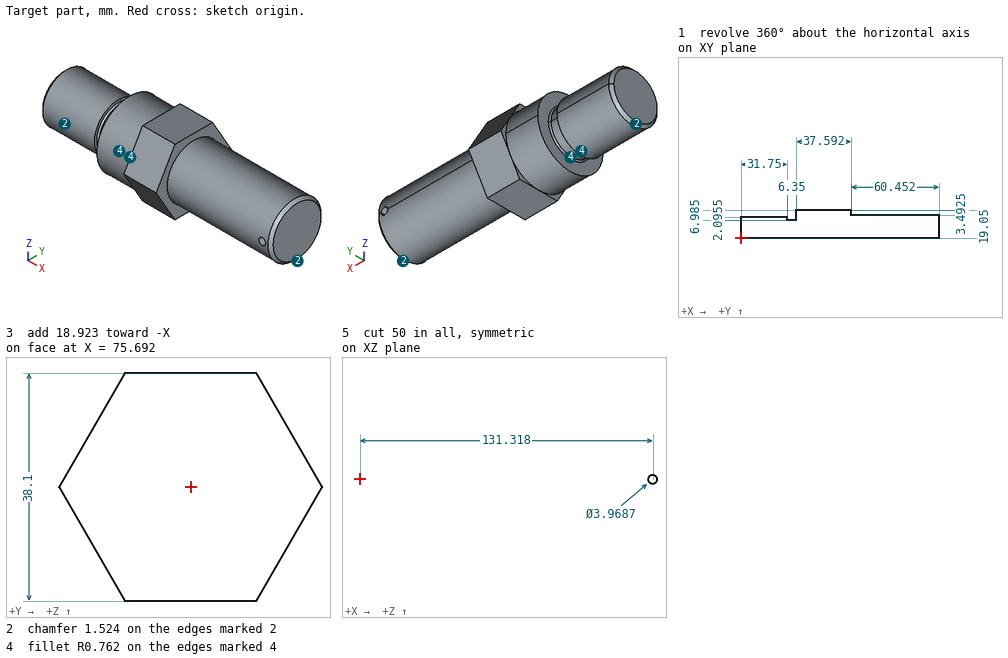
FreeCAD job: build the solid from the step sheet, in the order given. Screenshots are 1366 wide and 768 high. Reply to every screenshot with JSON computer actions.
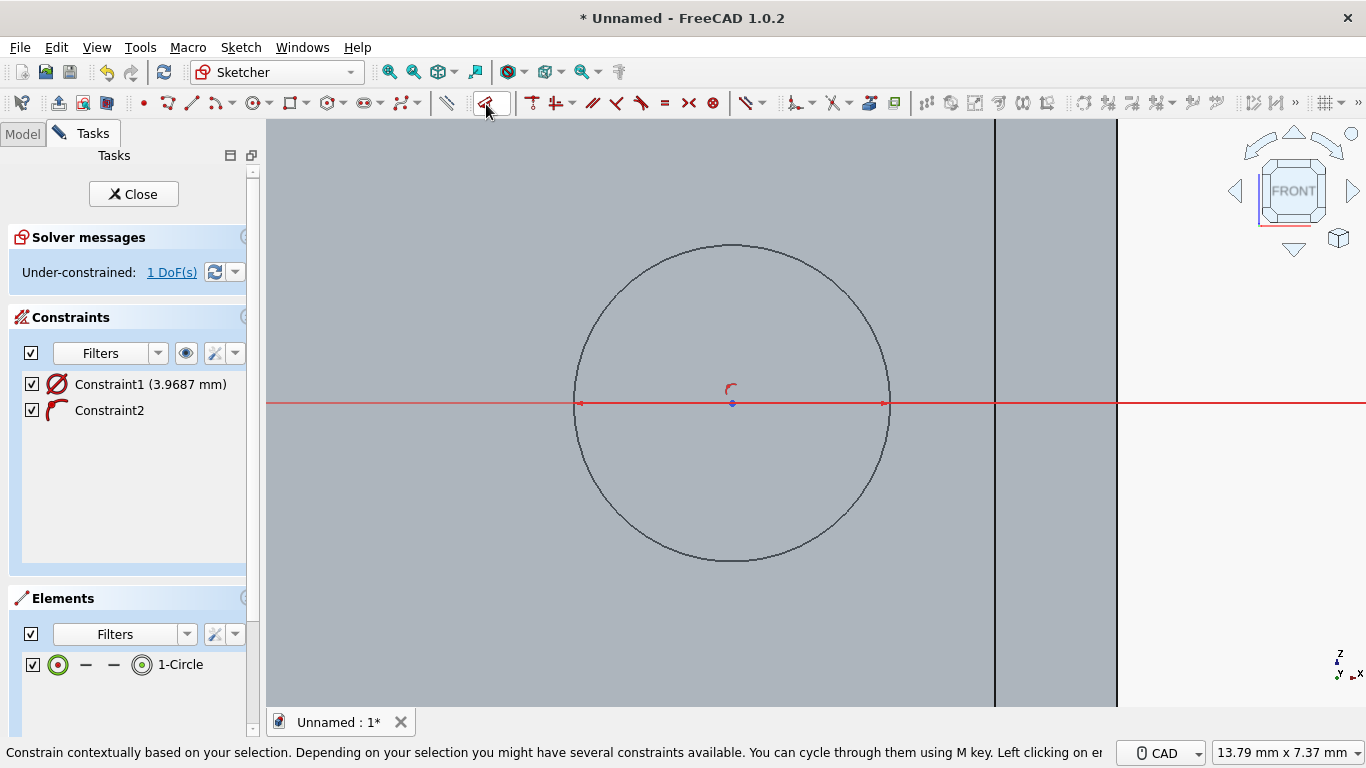
{"action": "left_click", "coordinate": [732, 403]}
{"action": "left_click", "coordinate": [513, 437]}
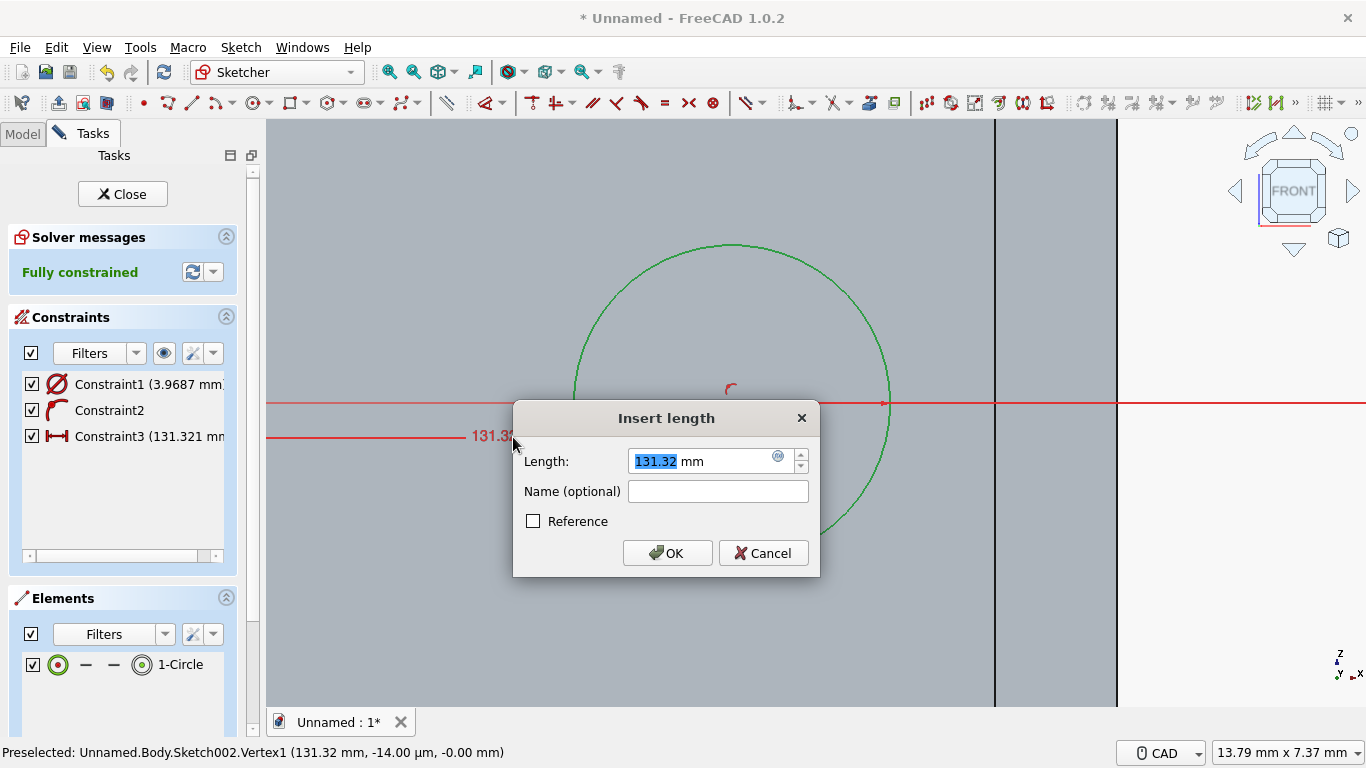
{"action": "type", "text": "131.318"}
{"action": "key", "text": "Return"}
{"action": "key", "text": "Escape"}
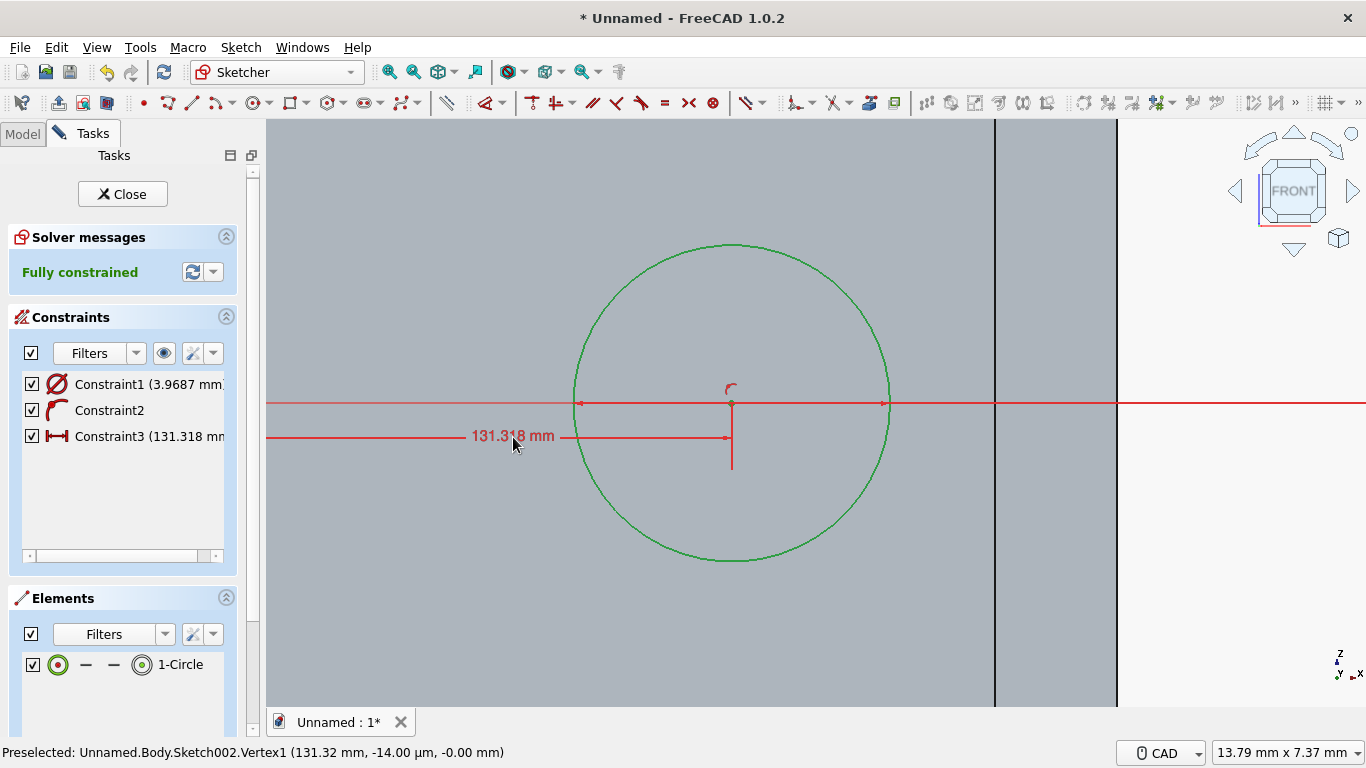
{"action": "left_click", "coordinate": [123, 194]}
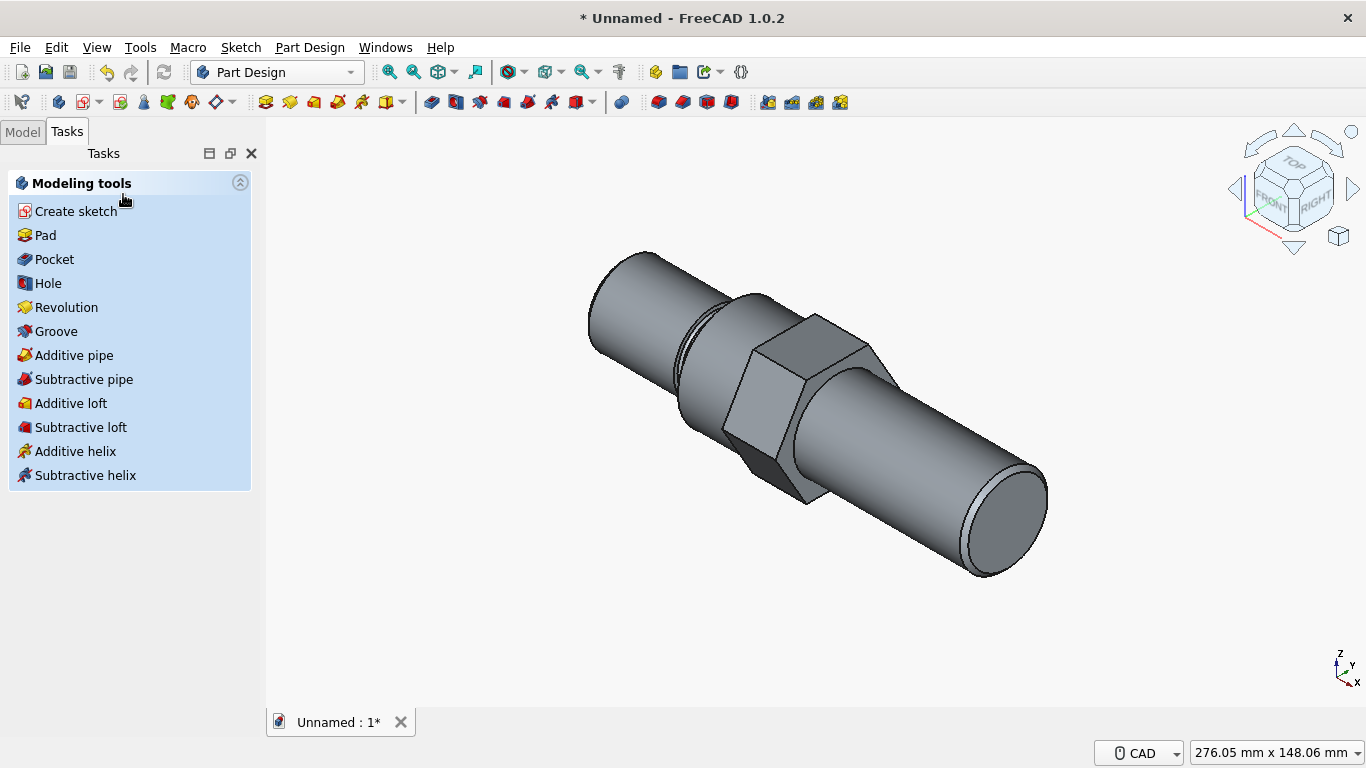
{"action": "left_click", "coordinate": [432, 102]}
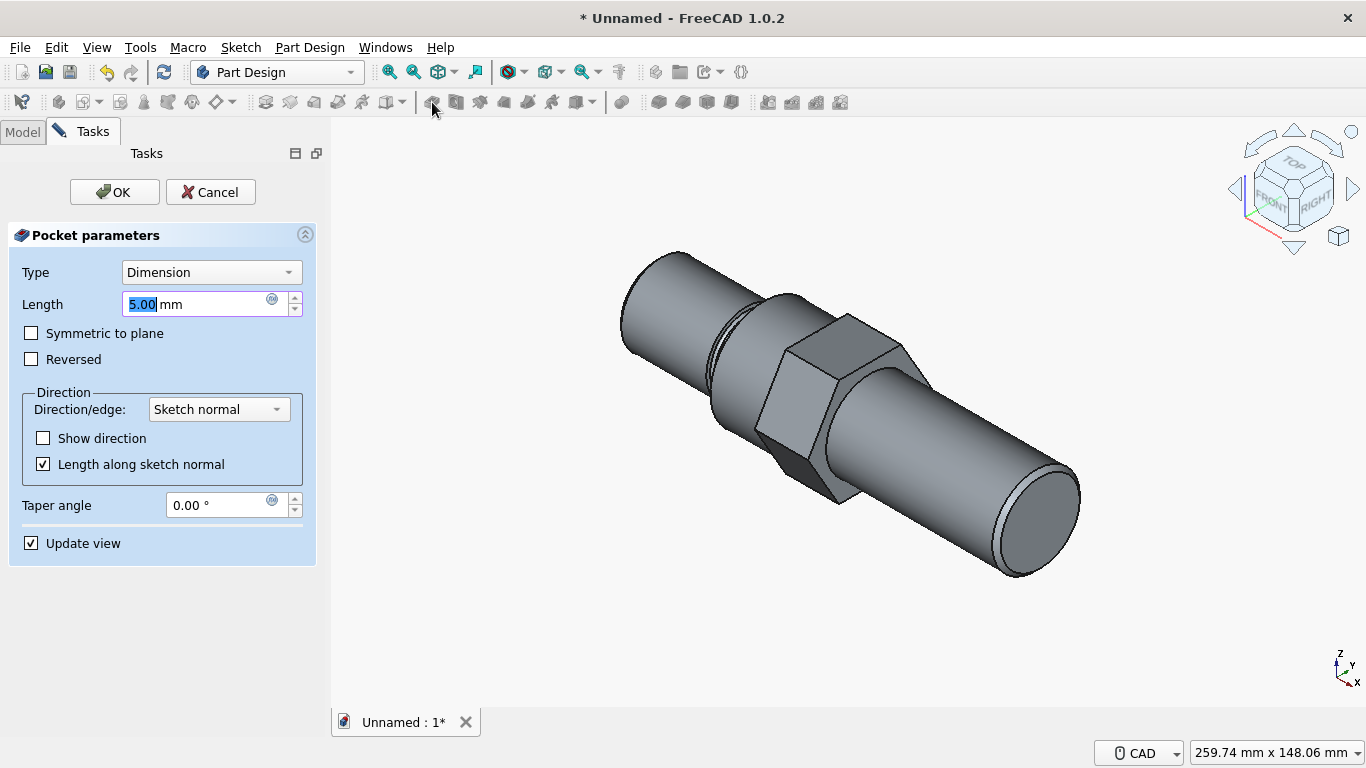
{"action": "type", "text": "50"}
{"action": "key", "text": "Tab"}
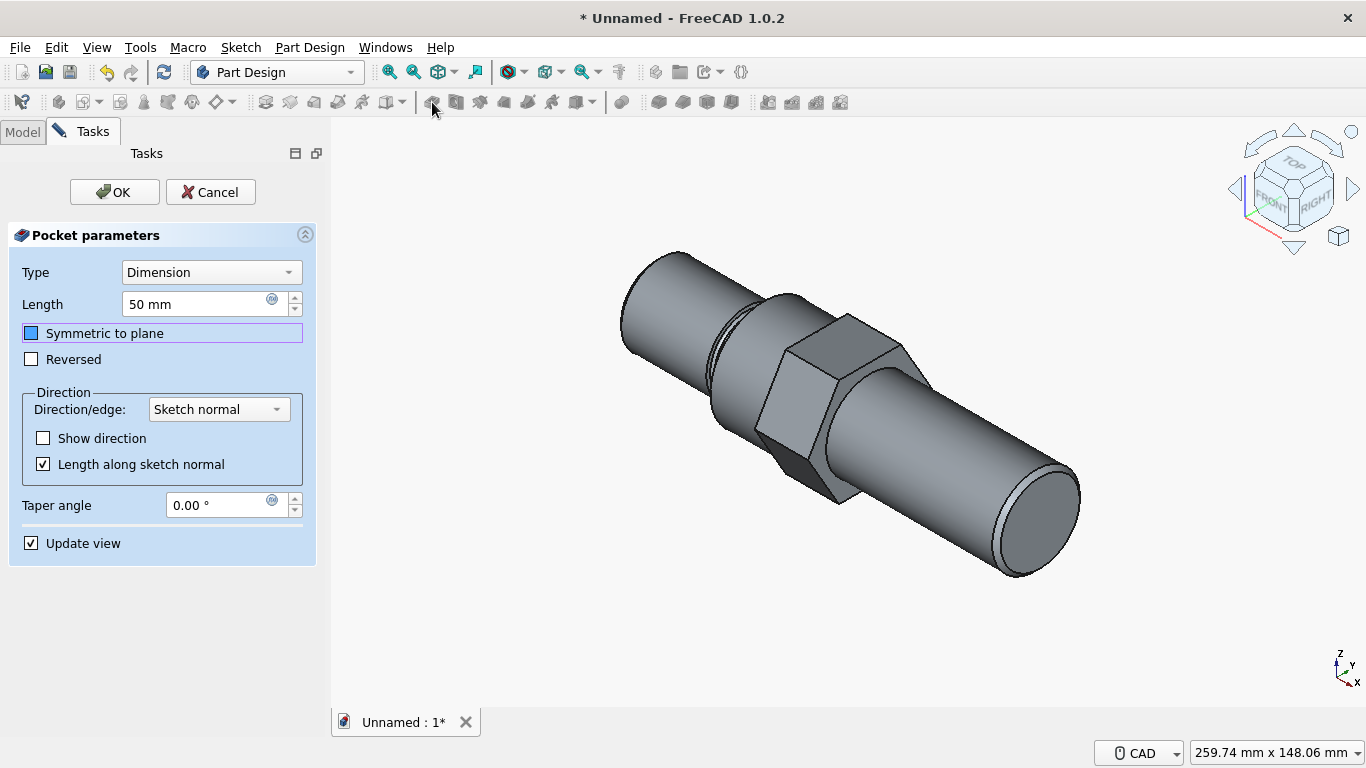
{"action": "left_click", "coordinate": [30, 333]}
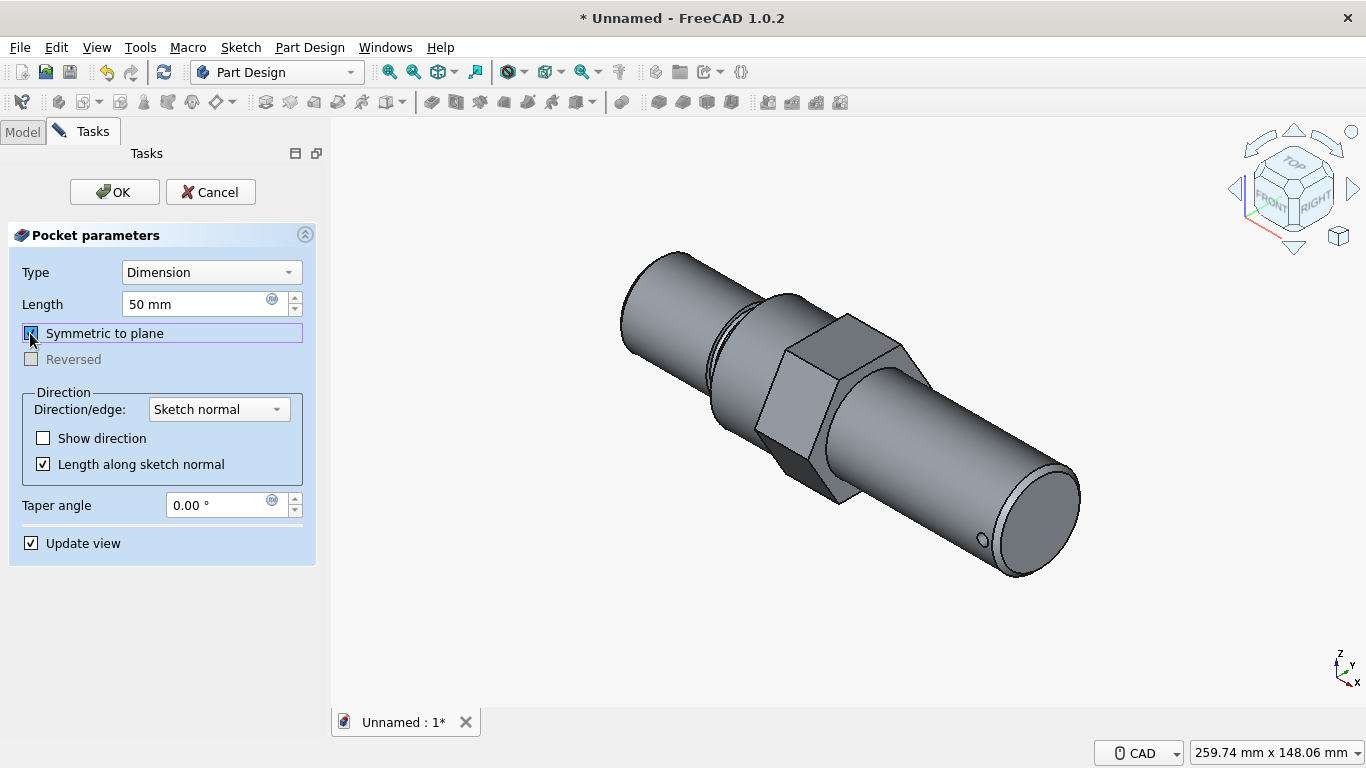
{"action": "left_click", "coordinate": [115, 192]}